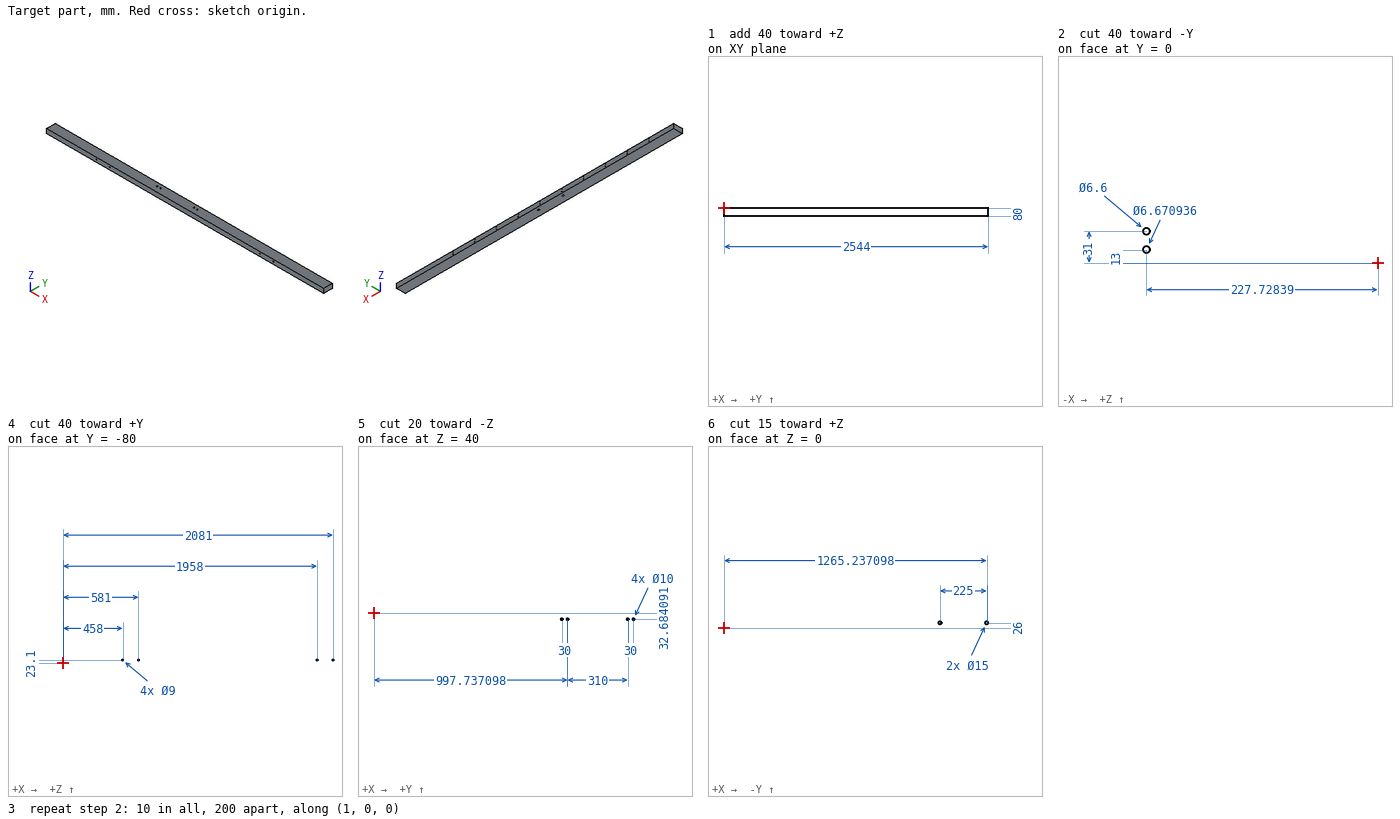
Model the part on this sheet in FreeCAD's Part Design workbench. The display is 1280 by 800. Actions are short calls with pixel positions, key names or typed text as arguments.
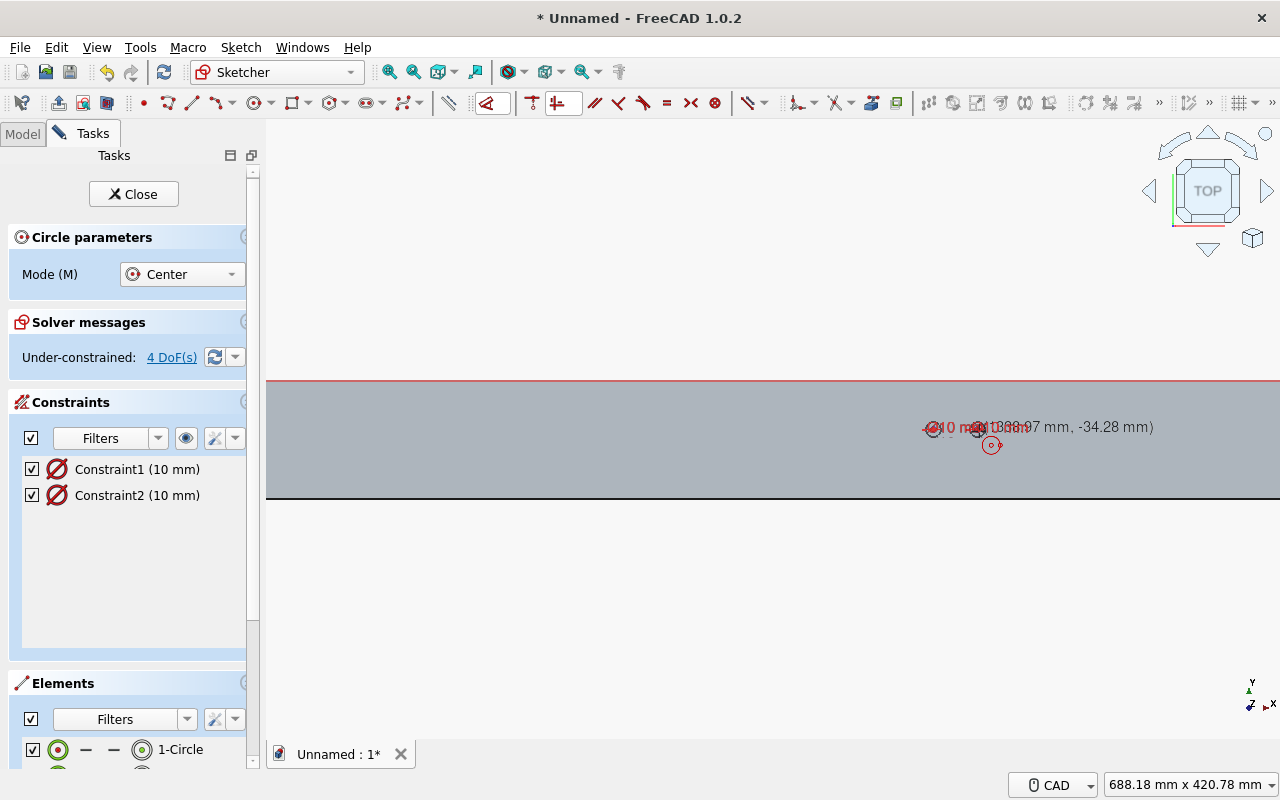
scroll(477, 429, up, 6)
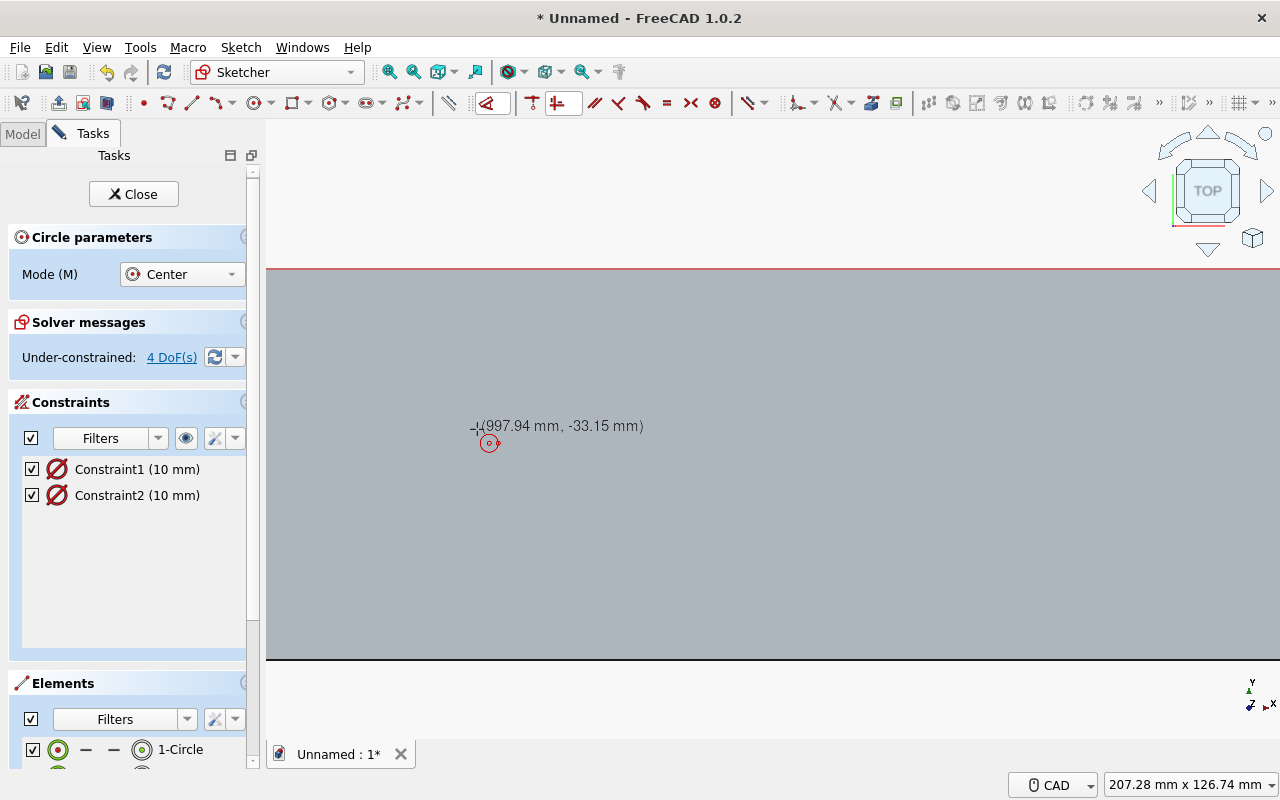
click(476, 429)
move(493, 412)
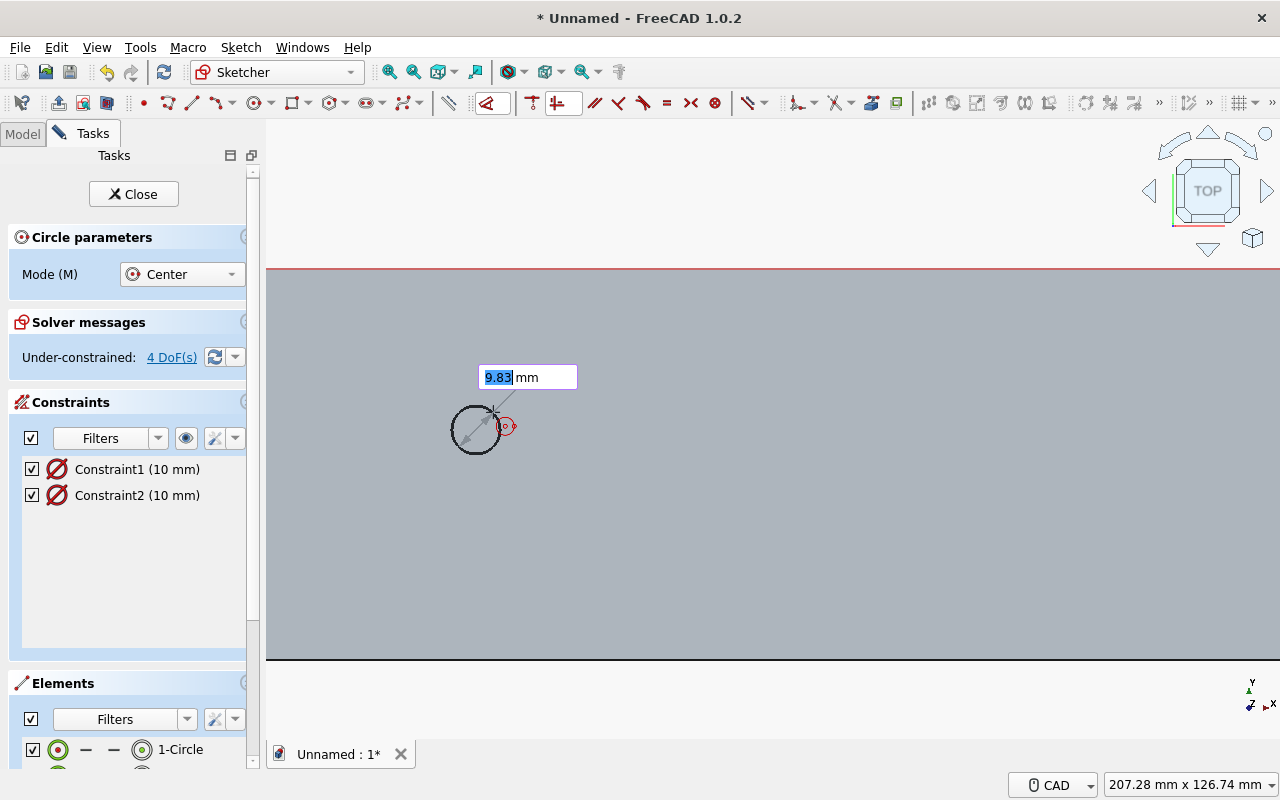
text(10)
key(Return)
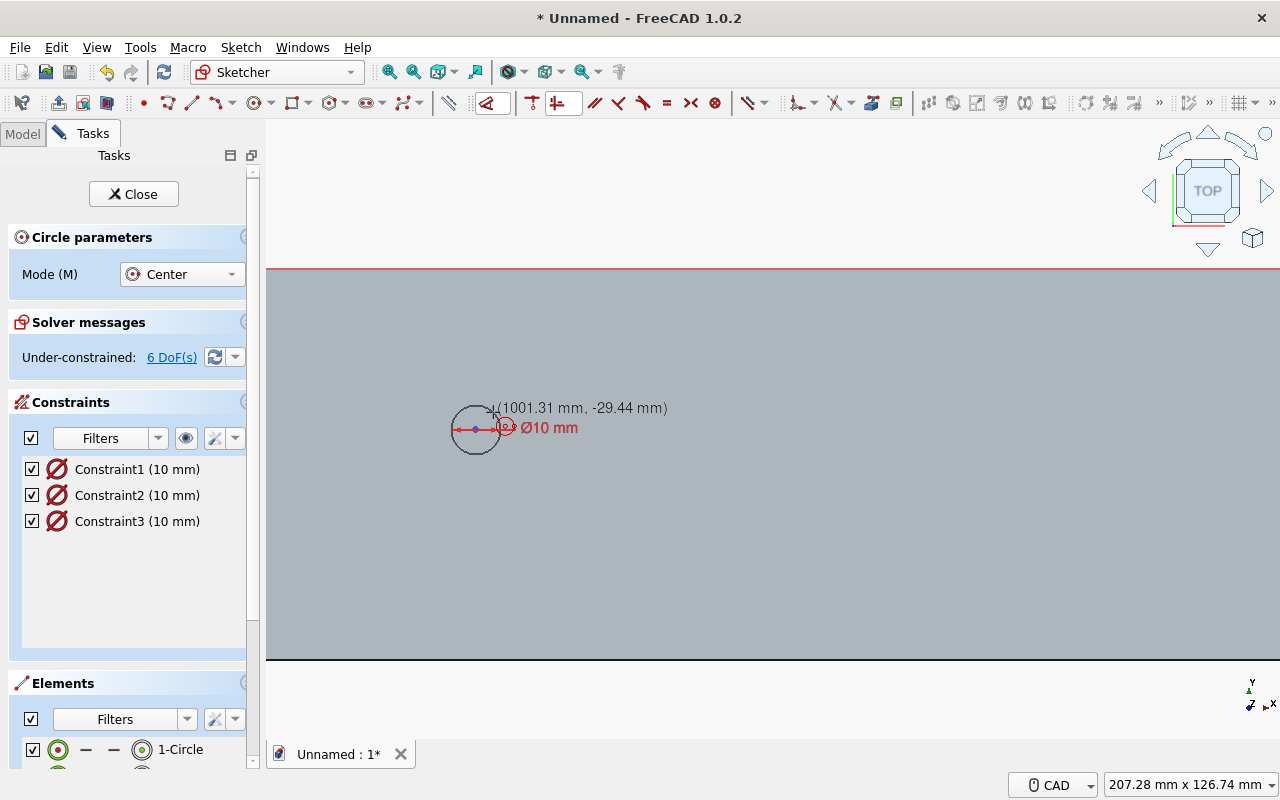
click(329, 429)
move(346, 412)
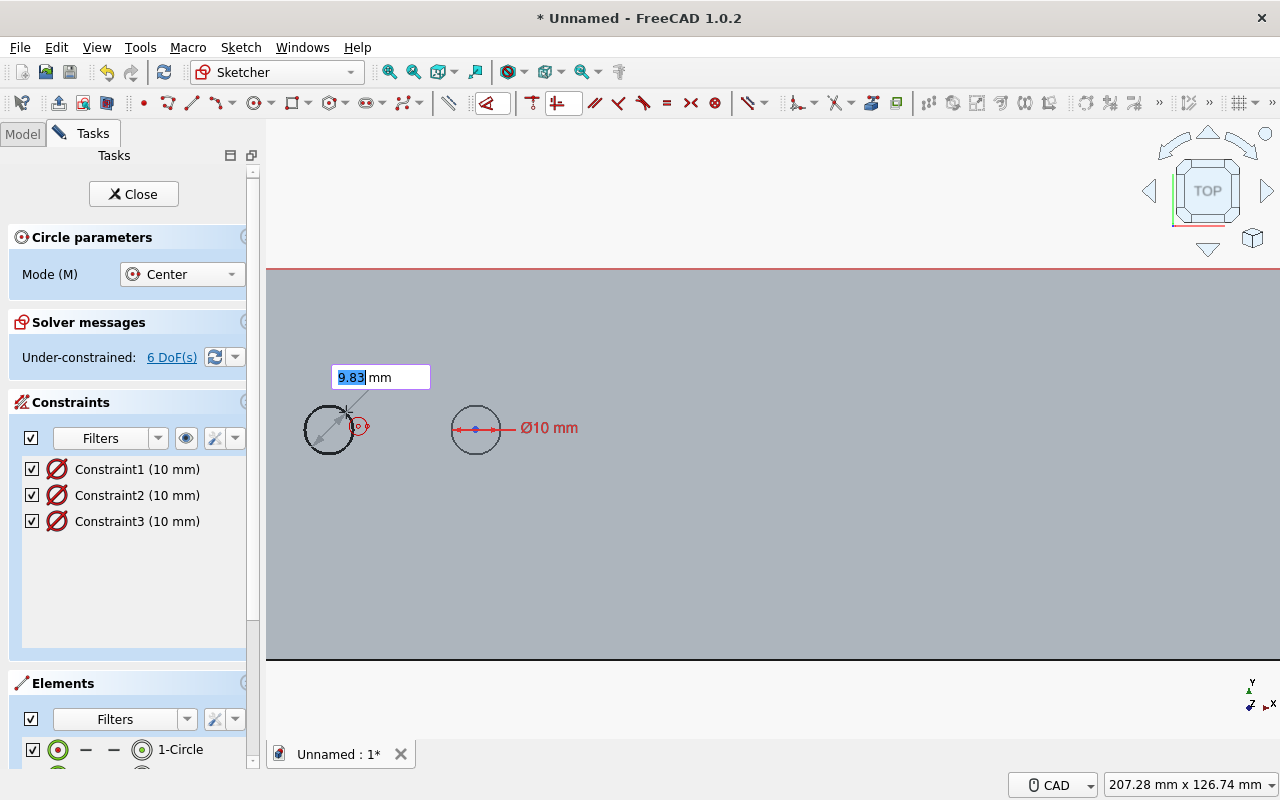
text(10)
key(Return)
key(Escape)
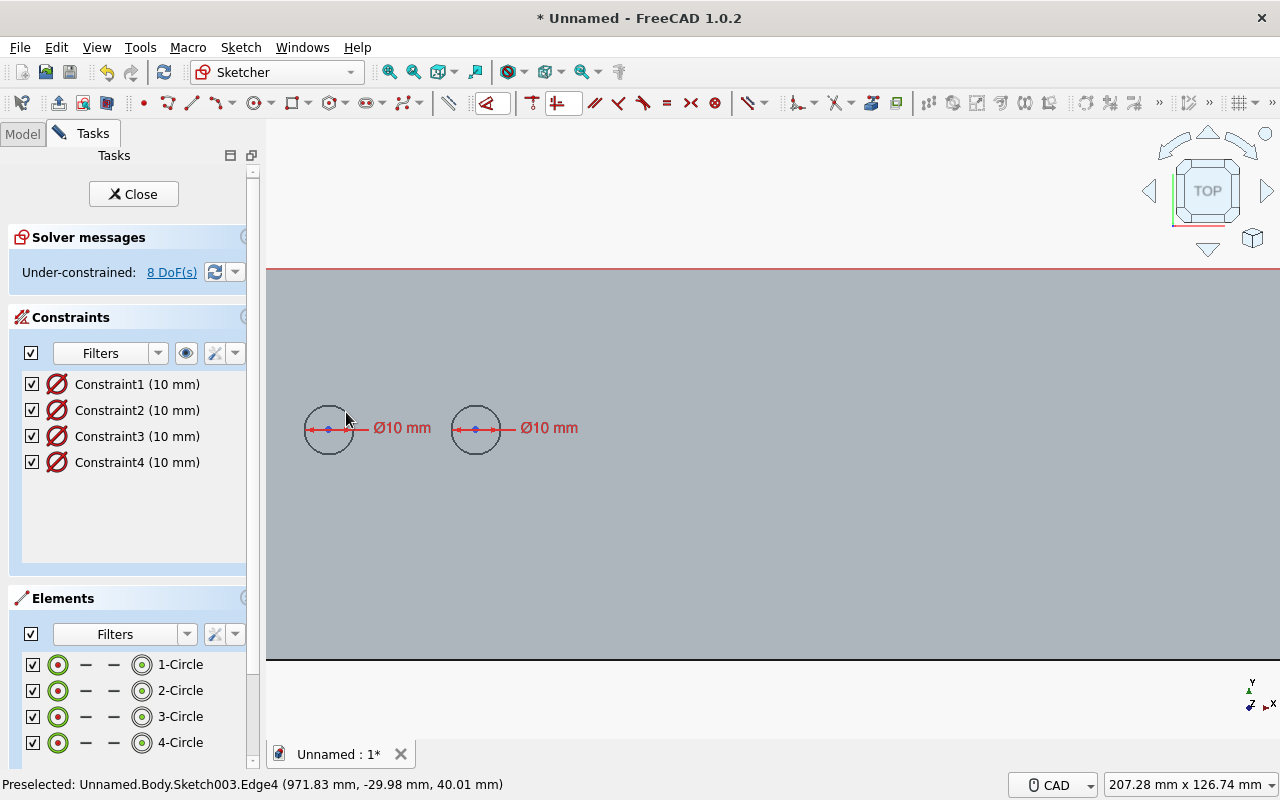
scroll(476, 429, down, 6)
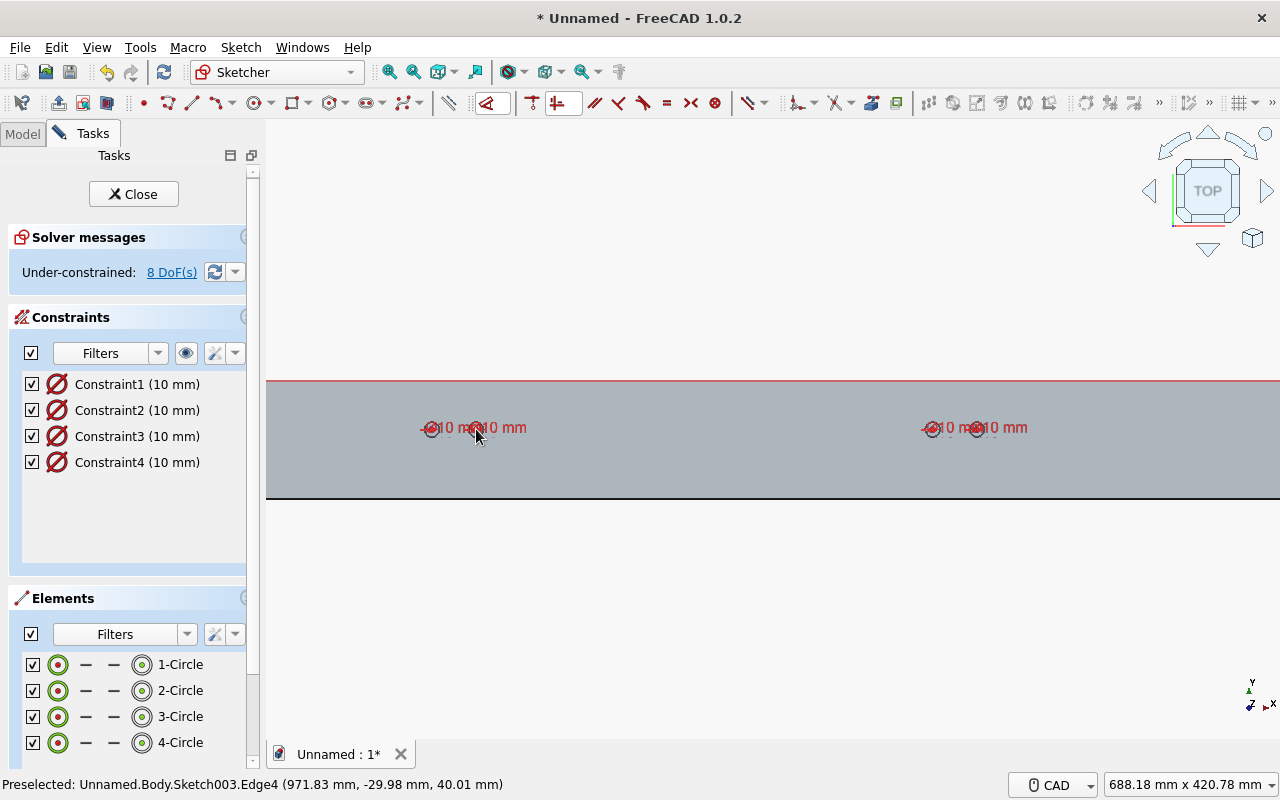
click(977, 430)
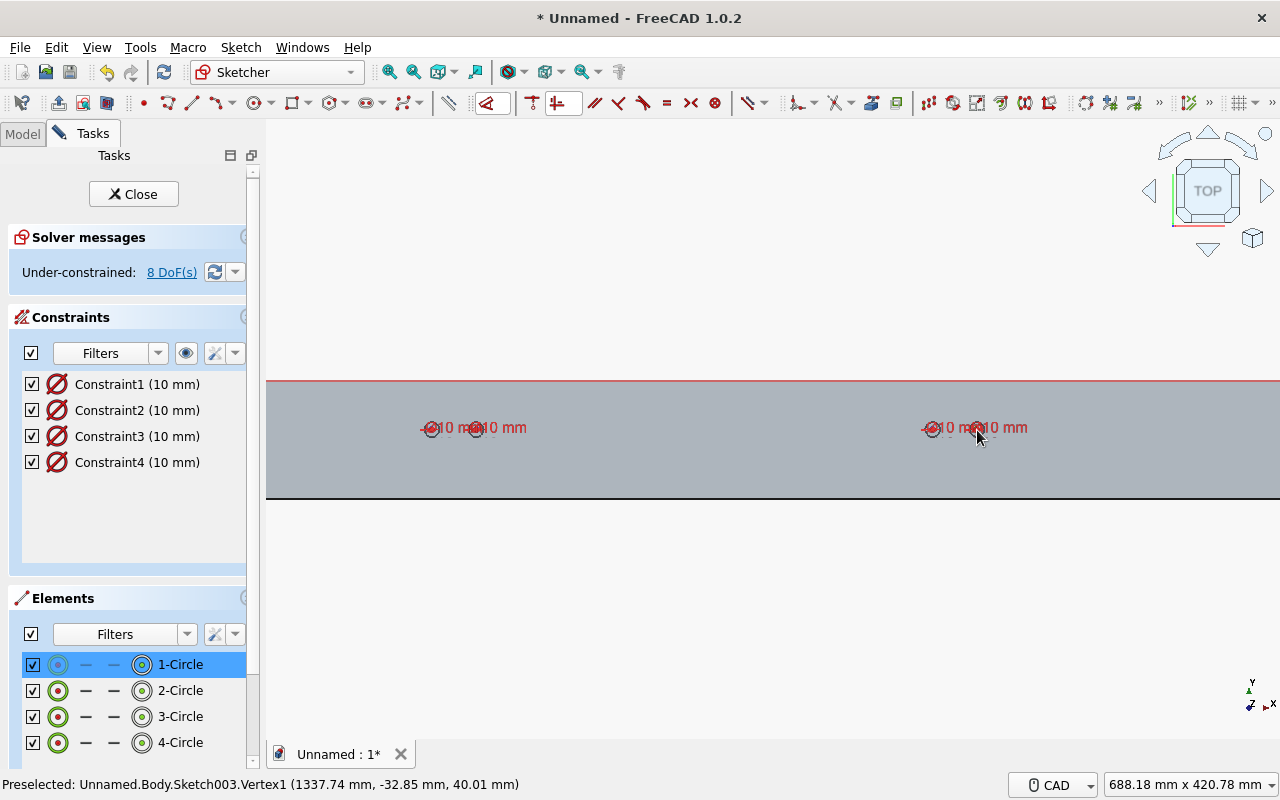
click(933, 430)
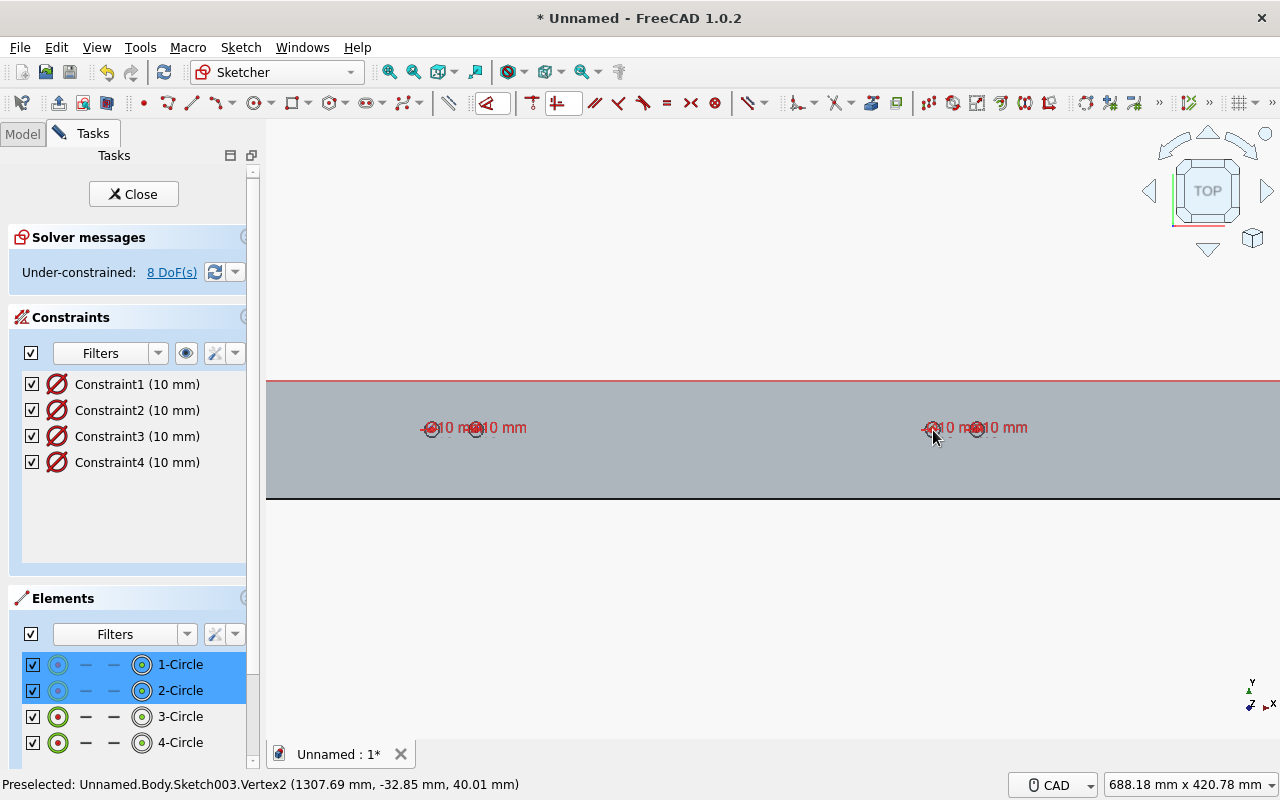
key(h)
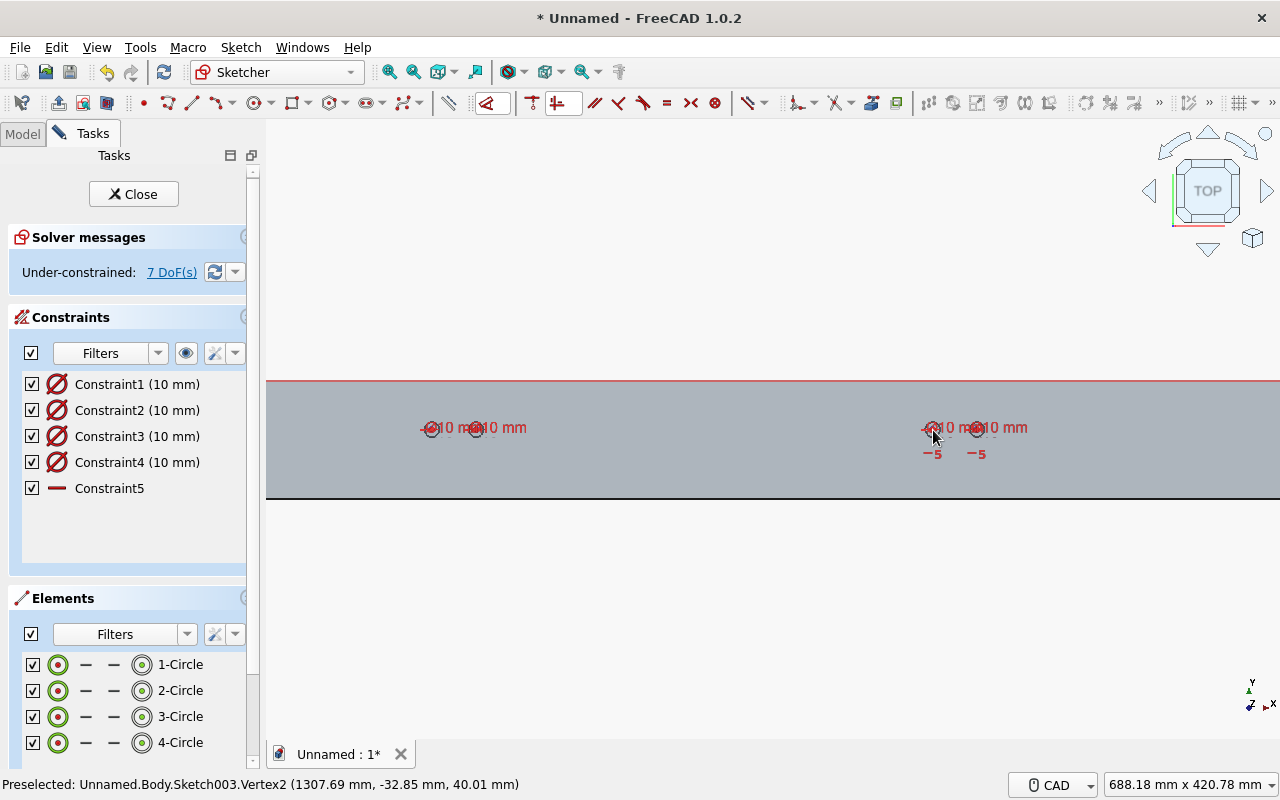
click(933, 430)